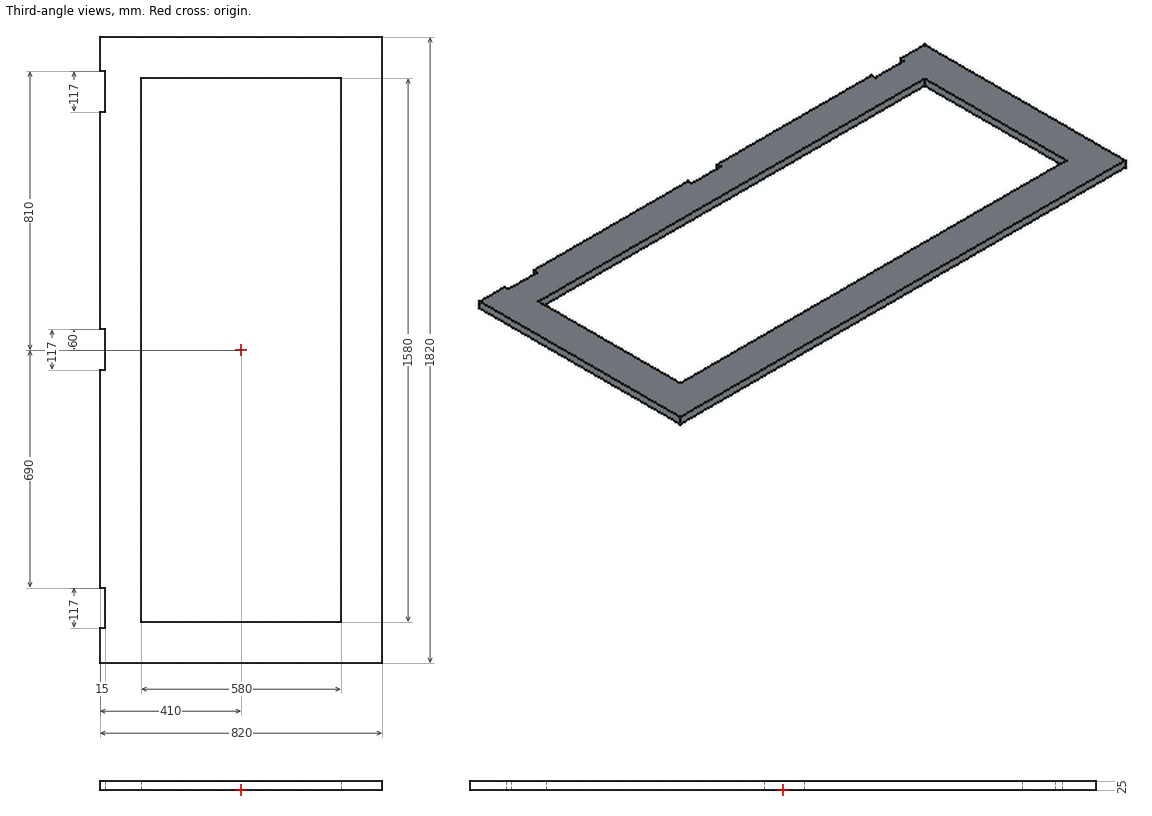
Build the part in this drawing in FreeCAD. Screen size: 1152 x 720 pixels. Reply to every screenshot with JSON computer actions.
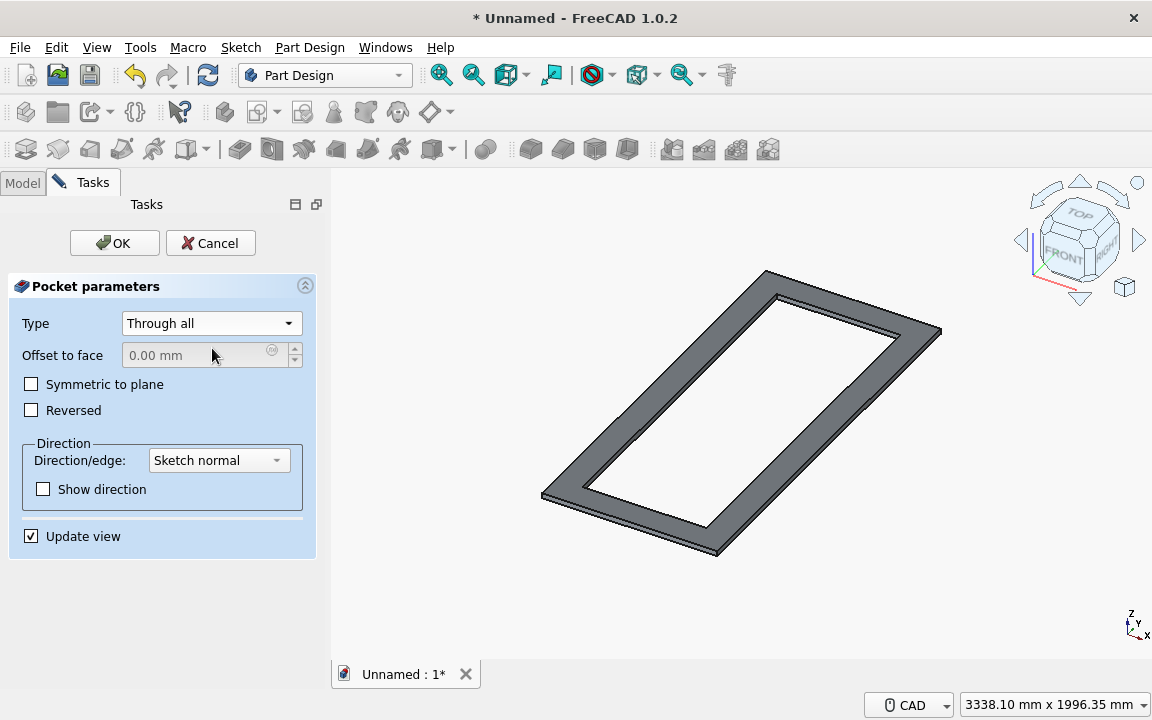
{"action": "left_click", "coordinate": [115, 243]}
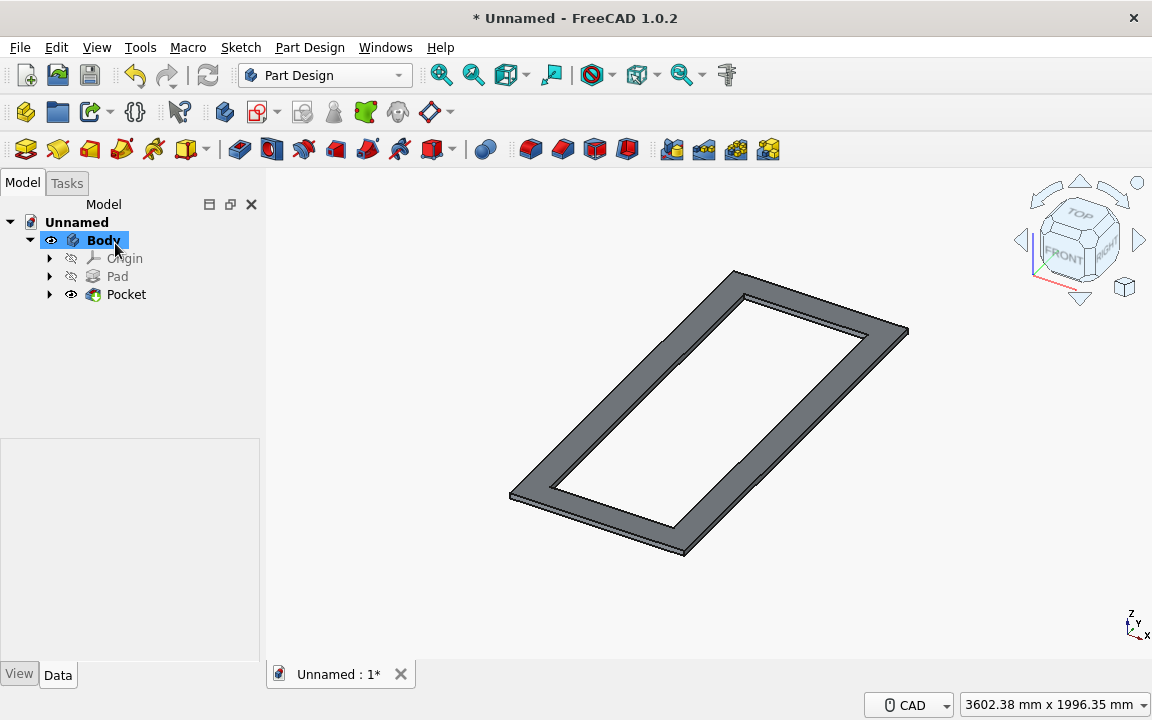
{"action": "left_click", "coordinate": [880, 339]}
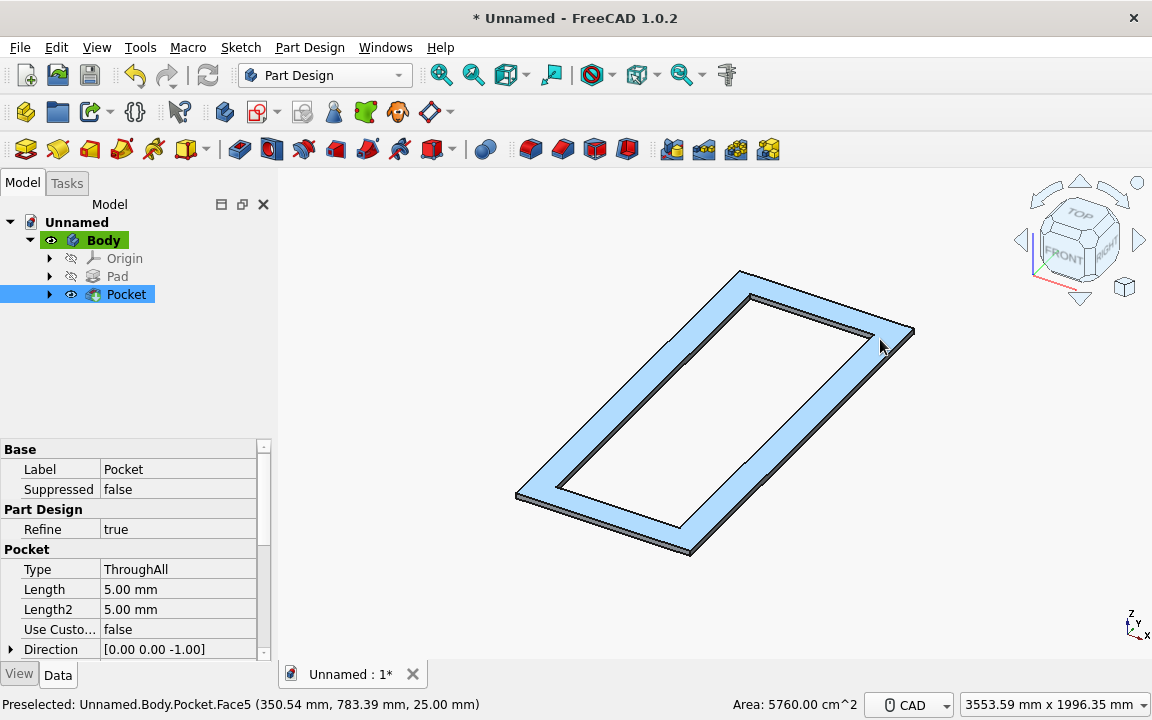
{"action": "left_click", "coordinate": [258, 112]}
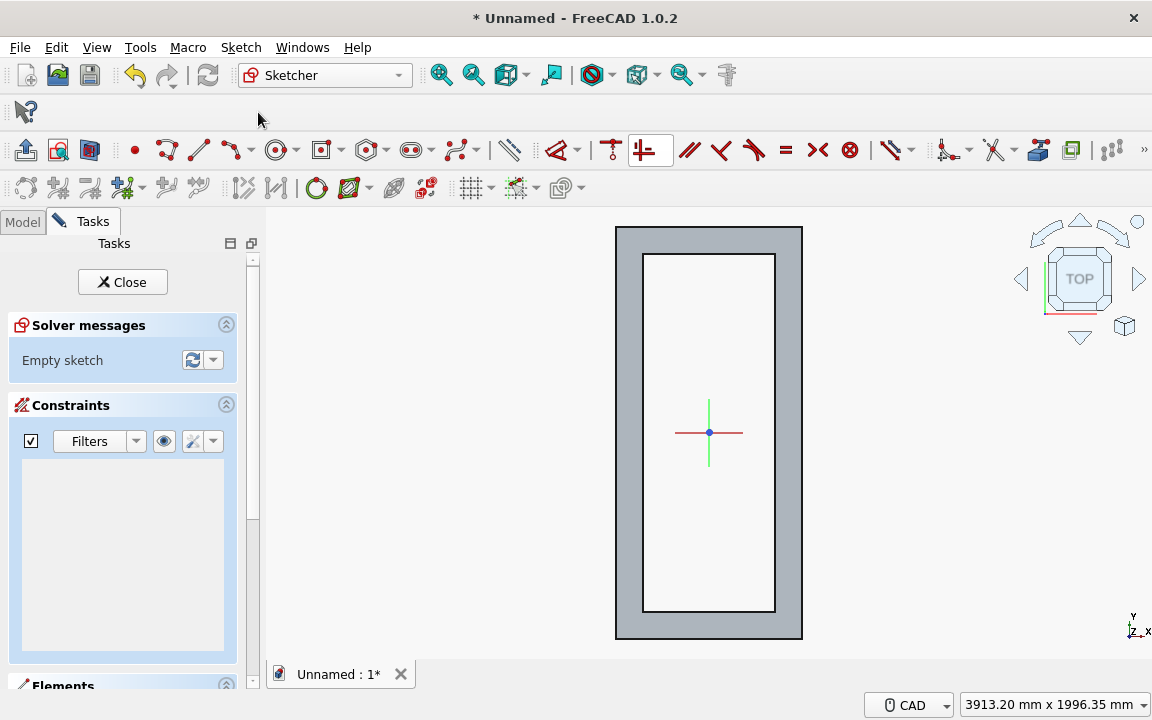
{"action": "scroll", "coordinate": [541, 435], "scroll_direction": "down", "scroll_amount": 1}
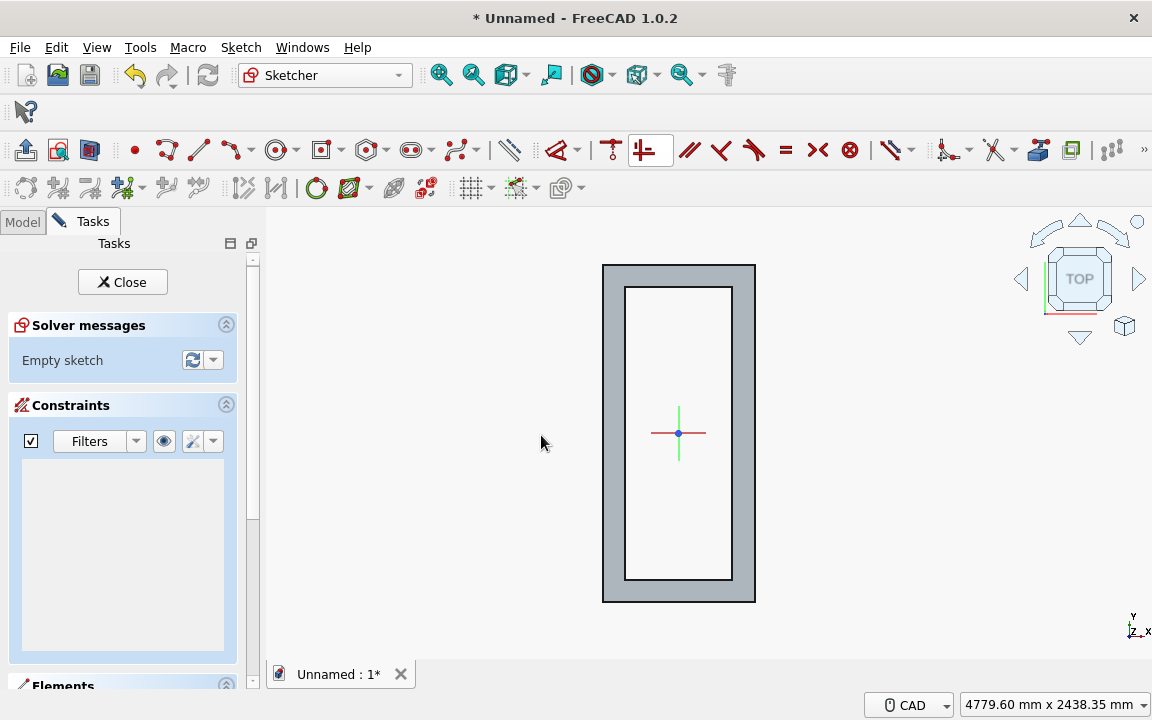
{"action": "left_click", "coordinate": [344, 150]}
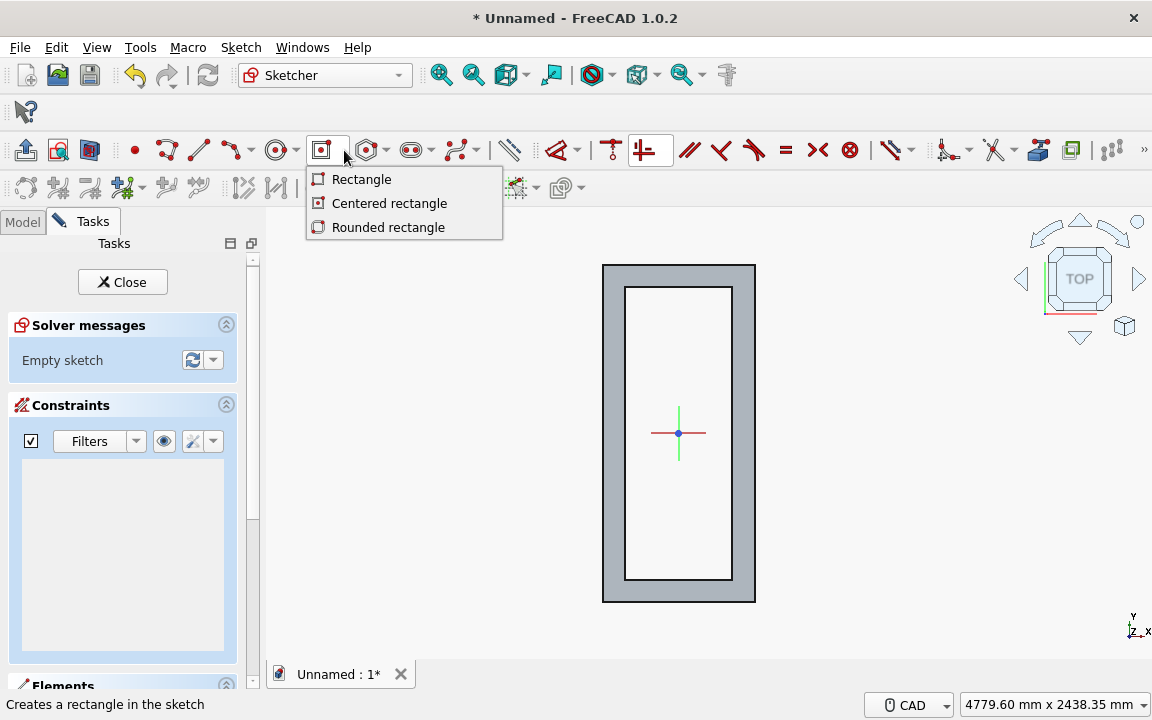
{"action": "left_click", "coordinate": [404, 179]}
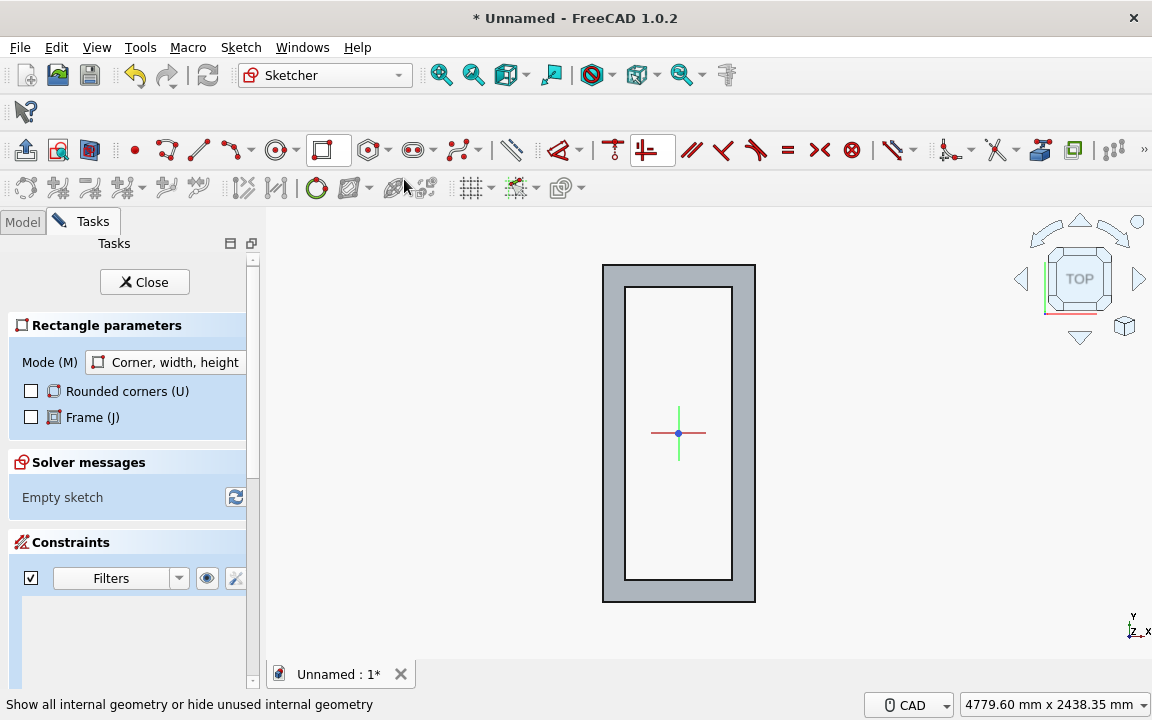
{"action": "scroll", "coordinate": [603, 561], "scroll_direction": "up", "scroll_amount": 9}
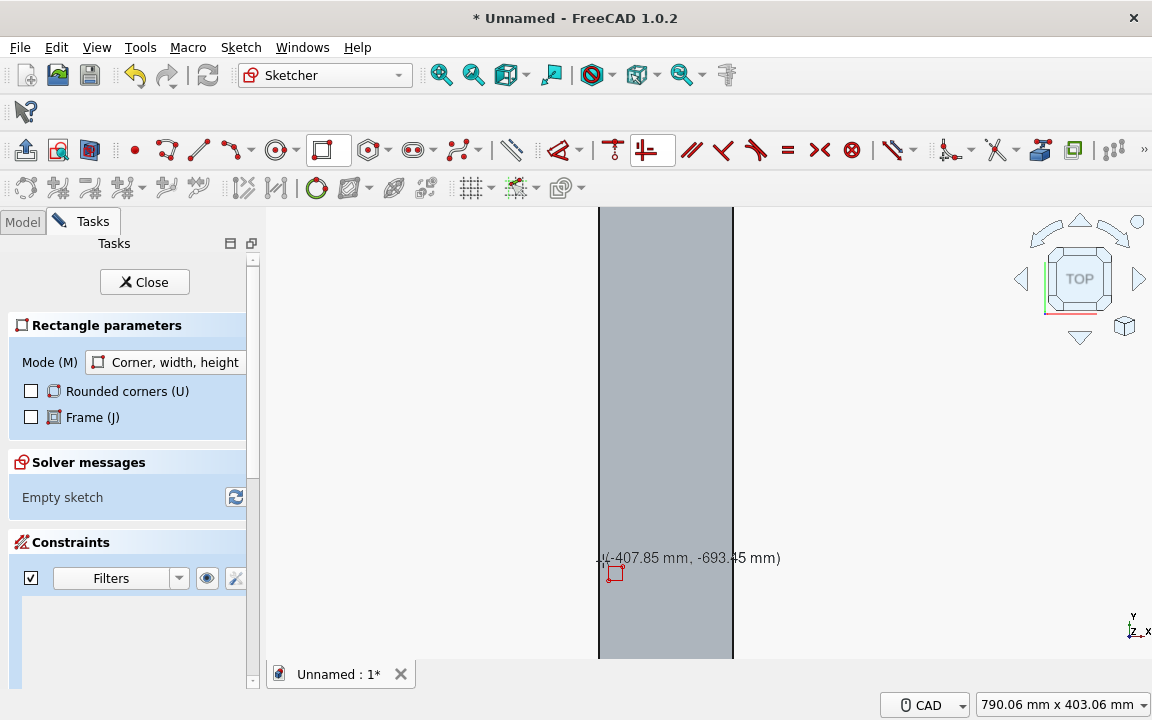
{"action": "scroll", "coordinate": [603, 562], "scroll_direction": "down", "scroll_amount": 9}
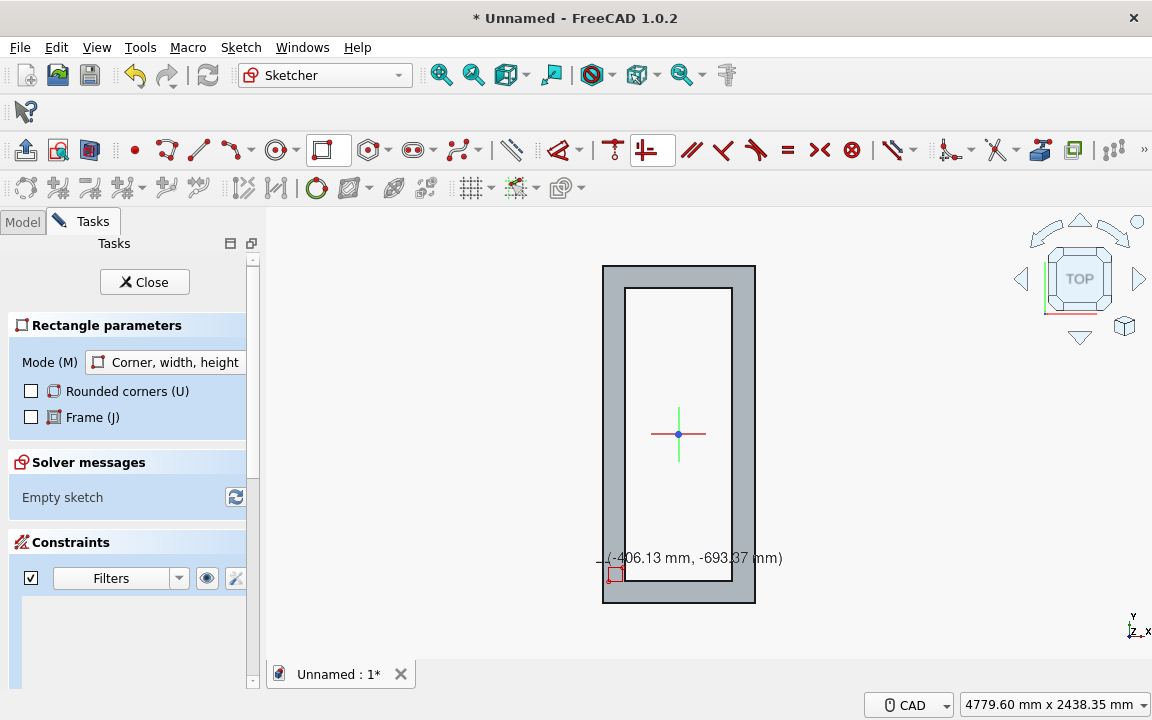
{"action": "left_click", "coordinate": [603, 562]}
{"action": "mouse_move", "coordinate": [605, 584]}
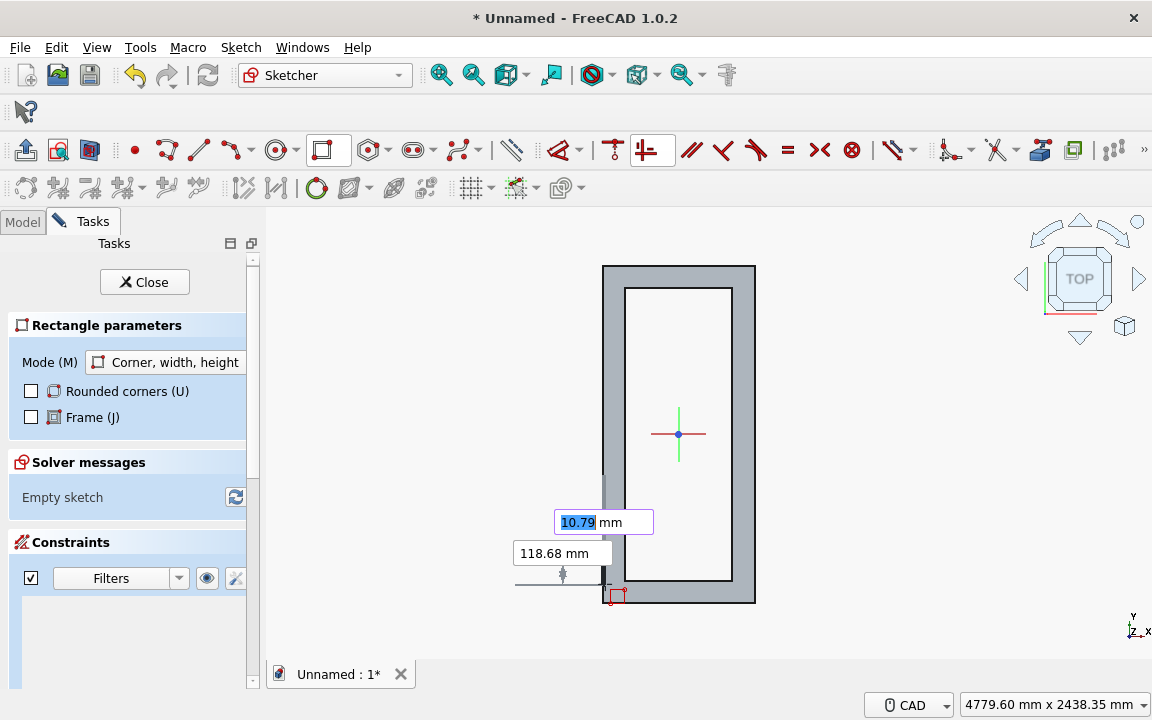
{"action": "type", "text": "15"}
{"action": "key", "text": "Tab"}
{"action": "type", "text": "117"}
{"action": "key", "text": "Return"}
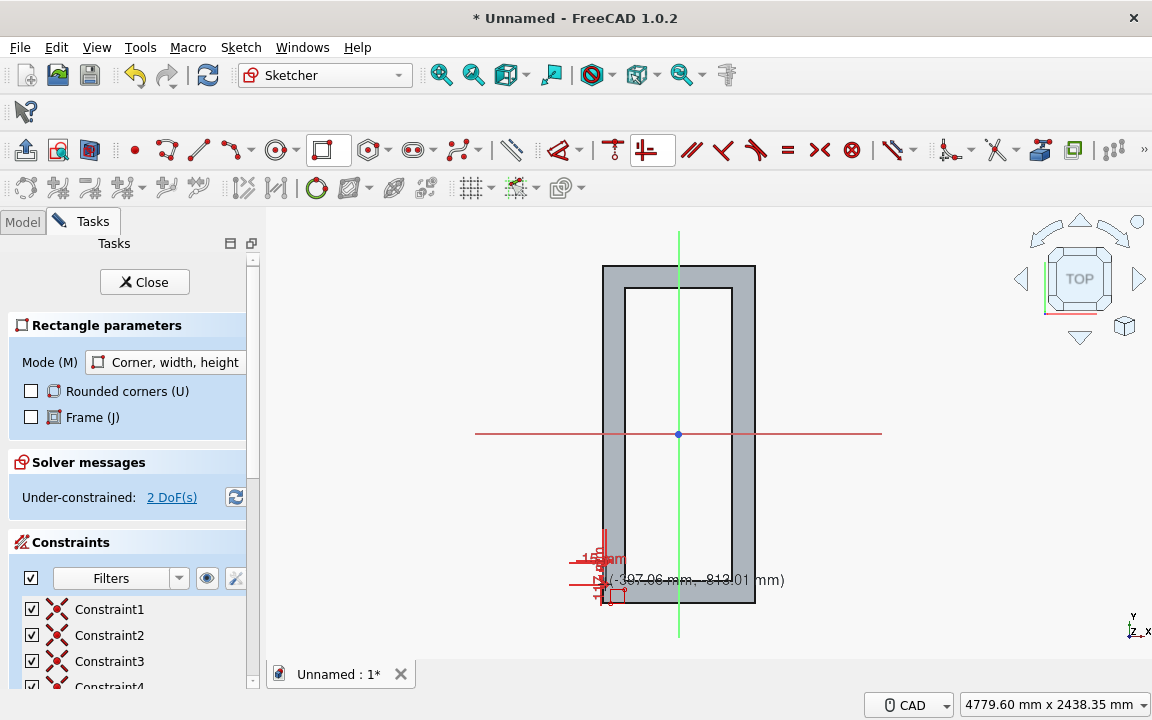
{"action": "scroll", "coordinate": [603, 423], "scroll_direction": "up", "scroll_amount": 9}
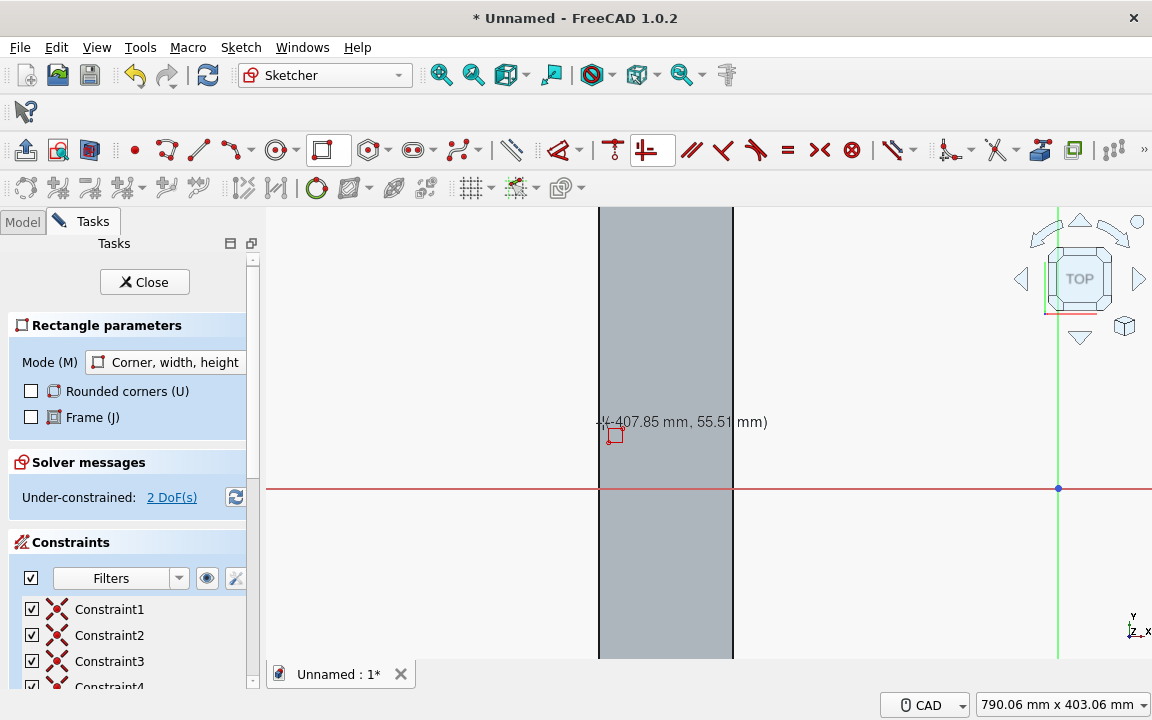
{"action": "scroll", "coordinate": [603, 422], "scroll_direction": "down", "scroll_amount": 9}